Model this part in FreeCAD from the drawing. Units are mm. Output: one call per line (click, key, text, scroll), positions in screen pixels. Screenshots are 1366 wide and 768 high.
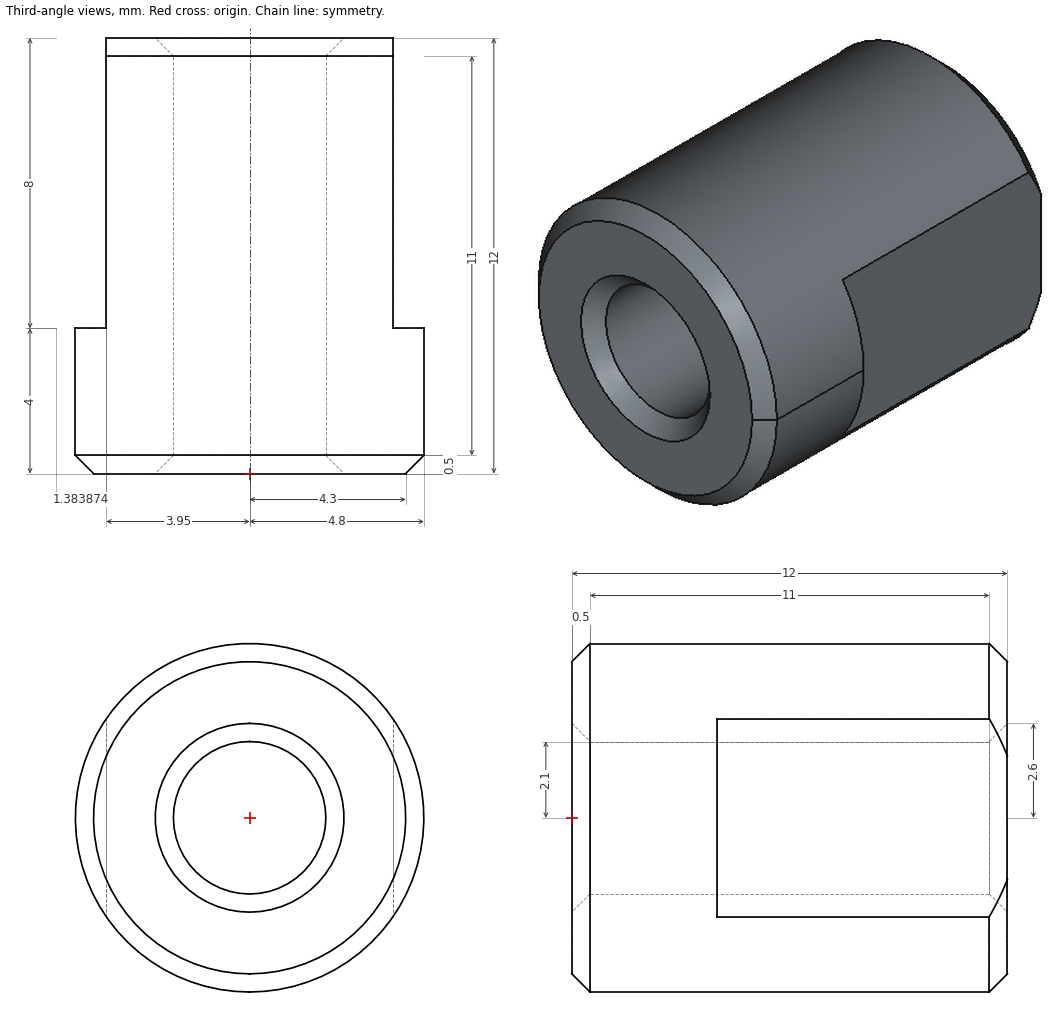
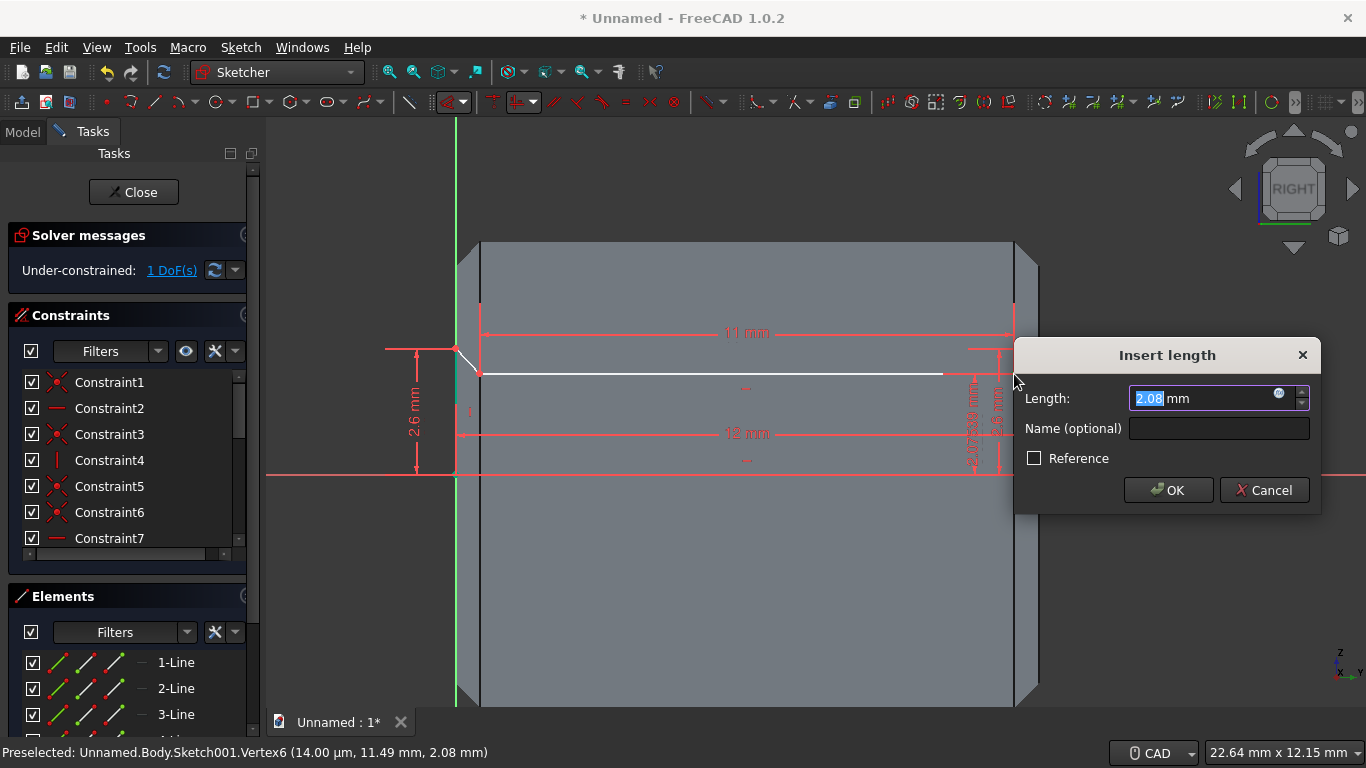
text(2.1)
key(Return)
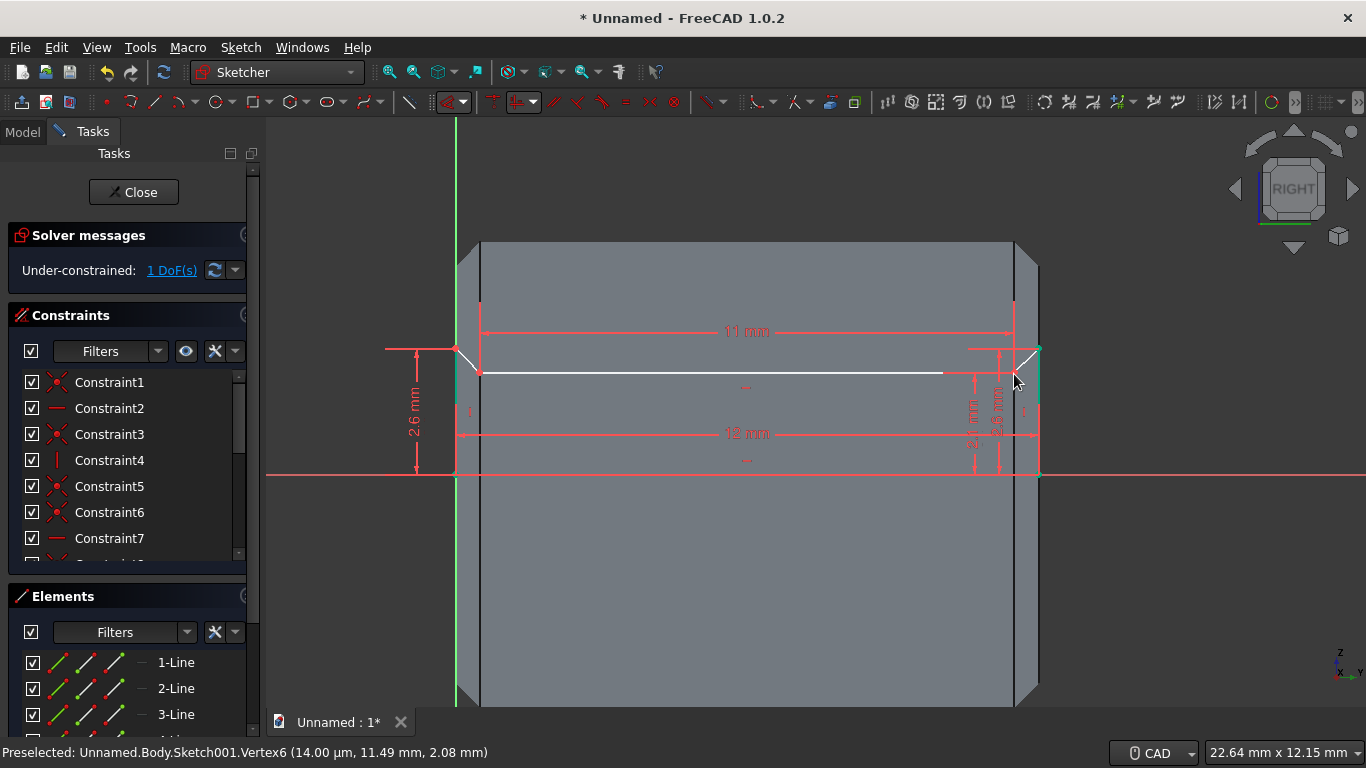
scroll(480, 373, up, 3)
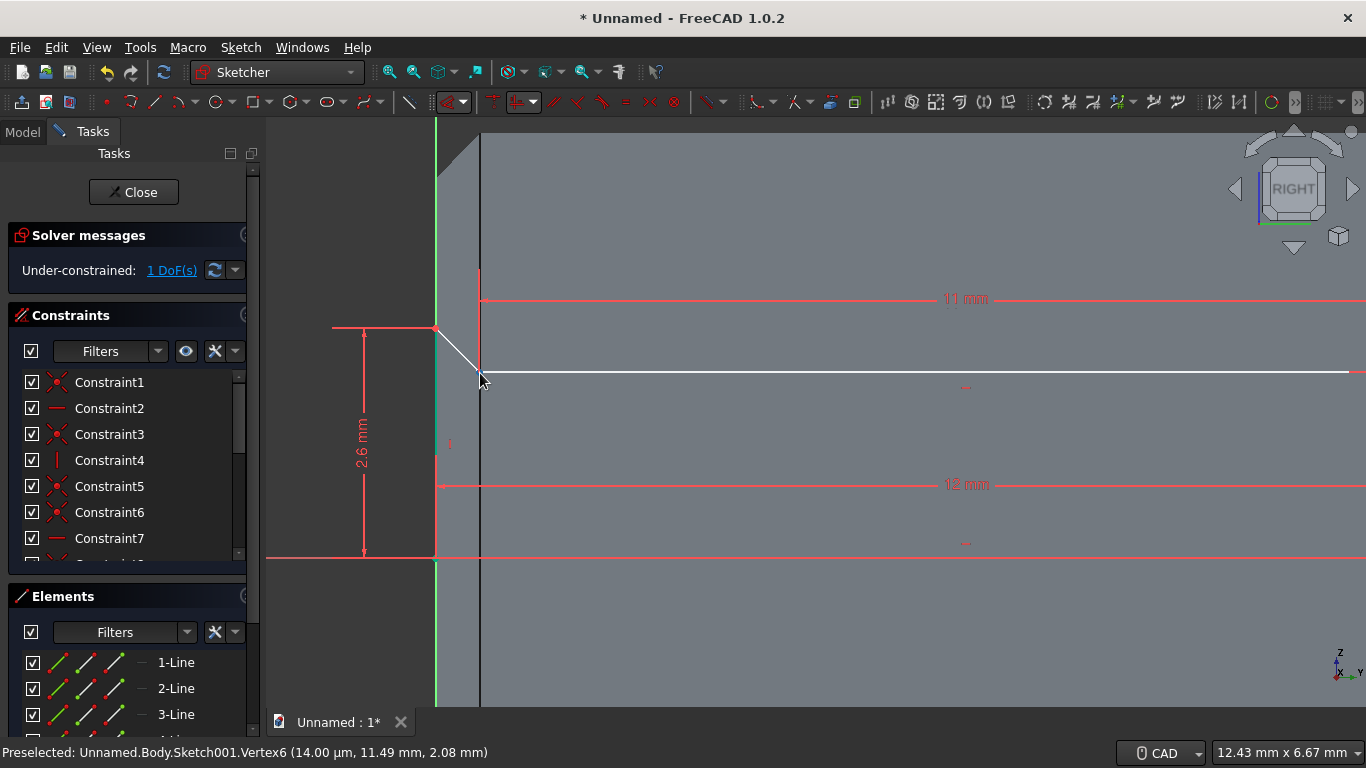
click(479, 372)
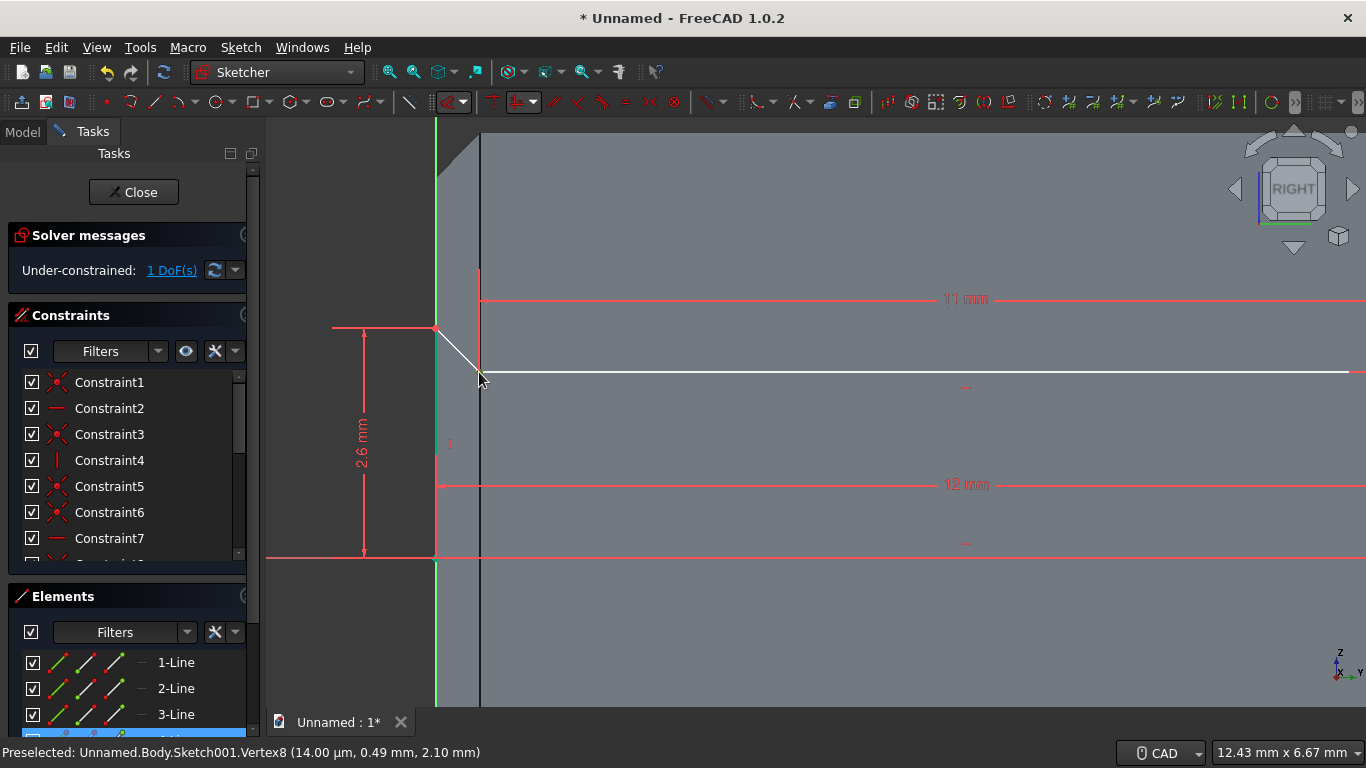
click(466, 102)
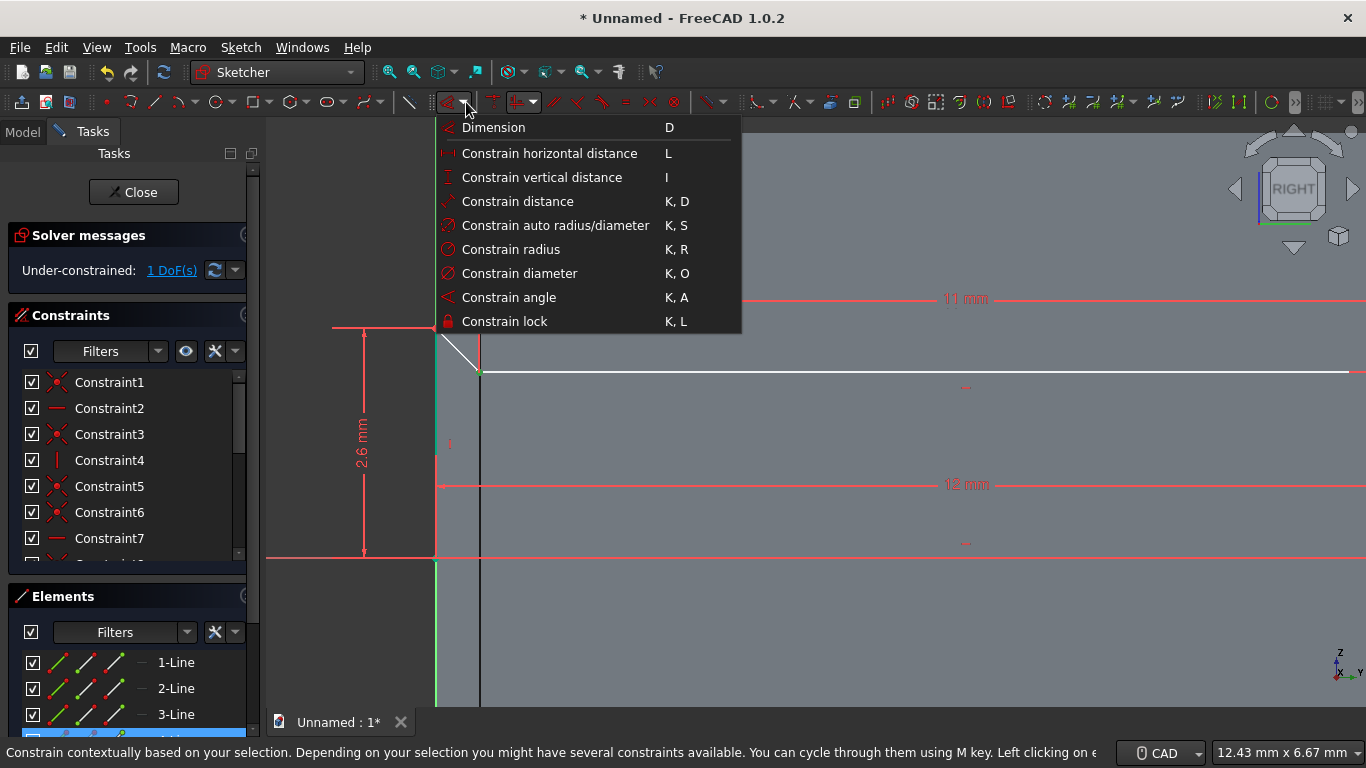
click(589, 153)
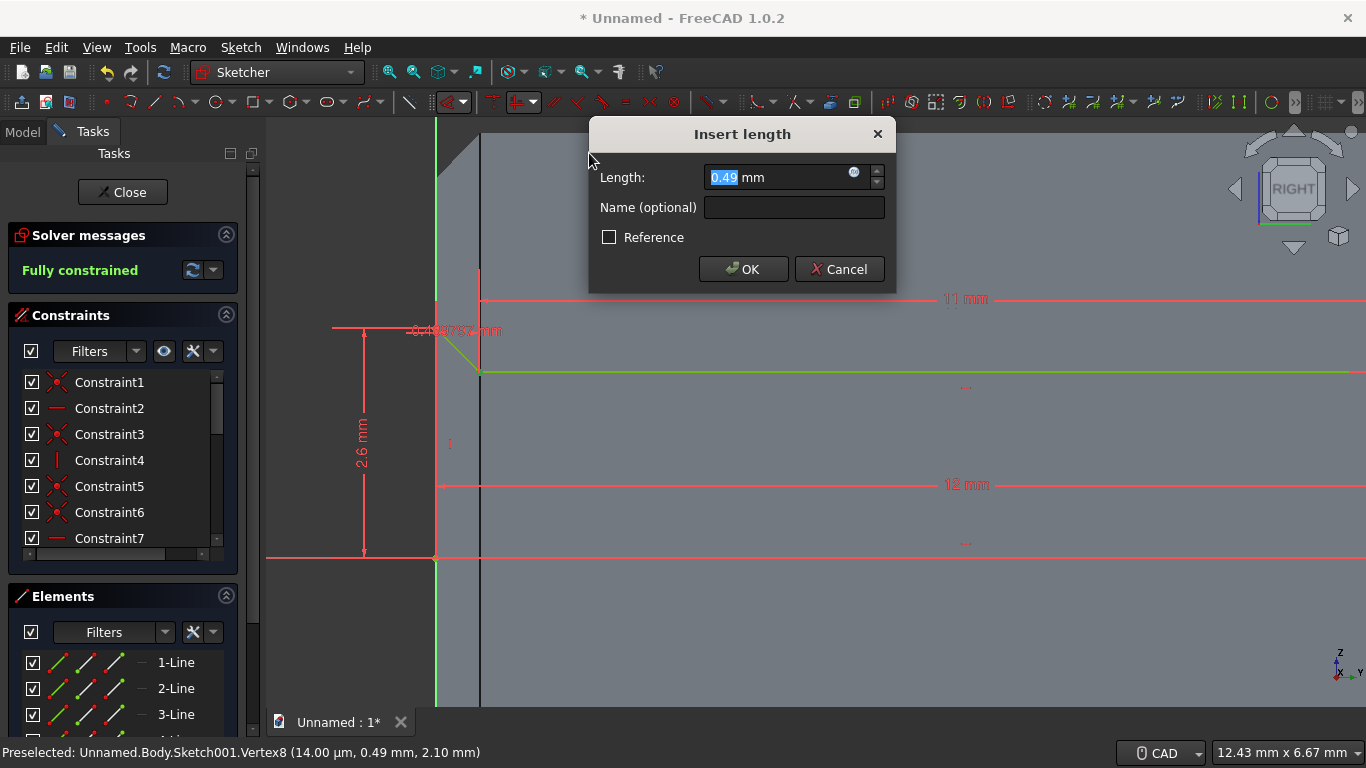
text(0.5)
key(Return)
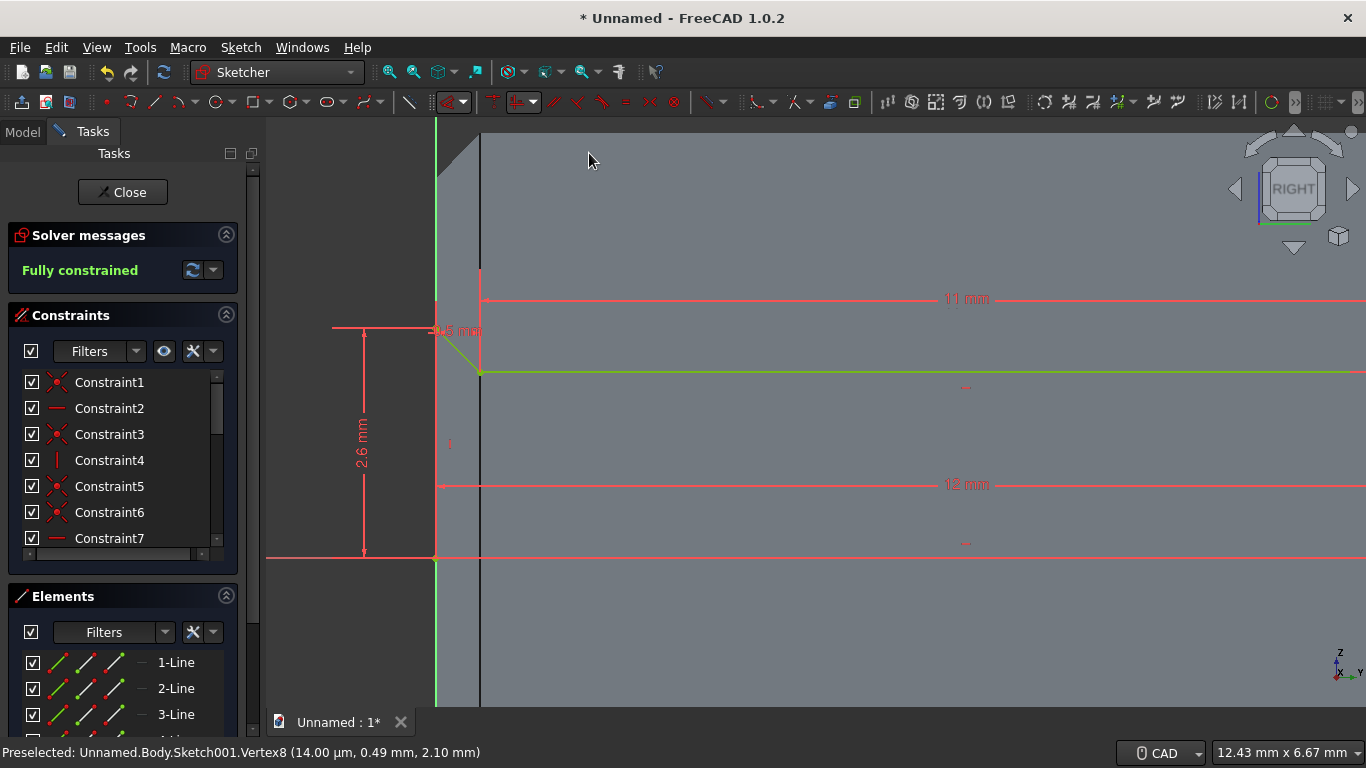
click(123, 192)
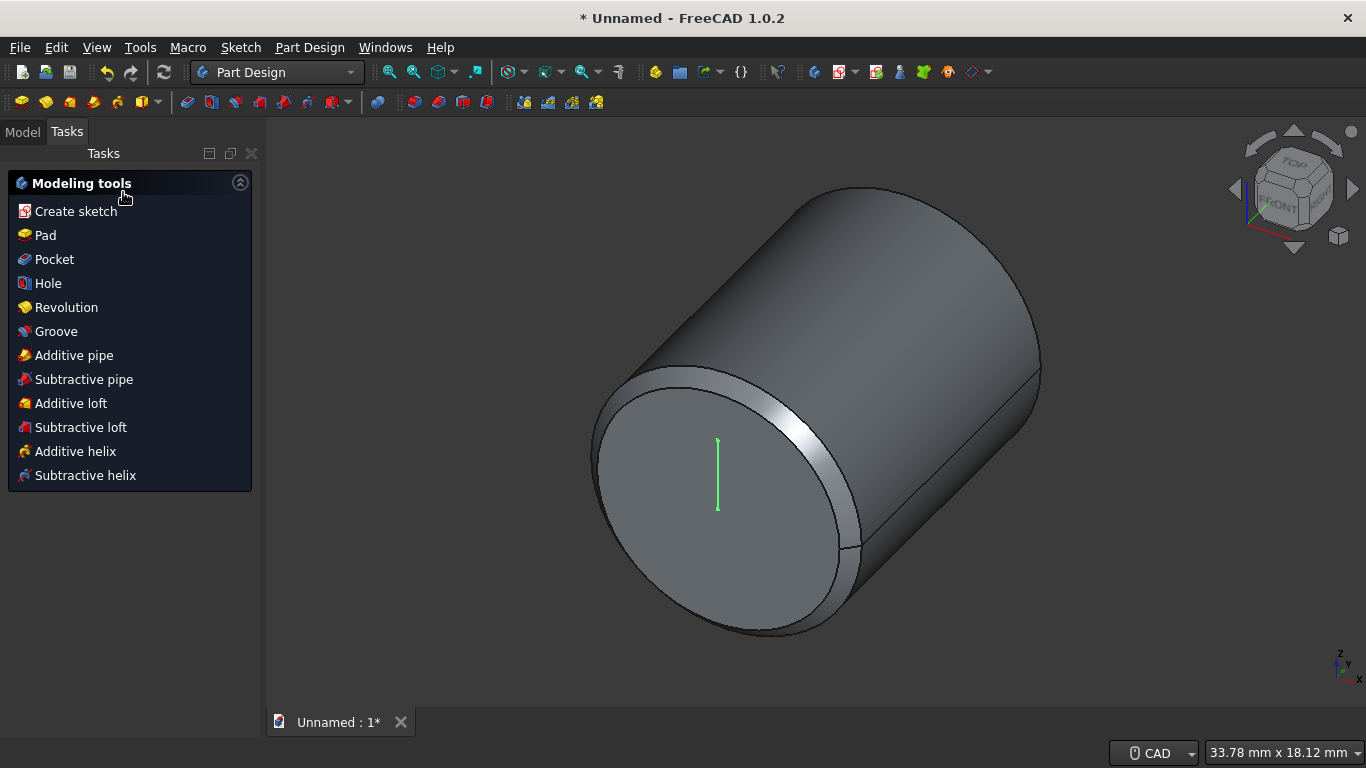
click(236, 102)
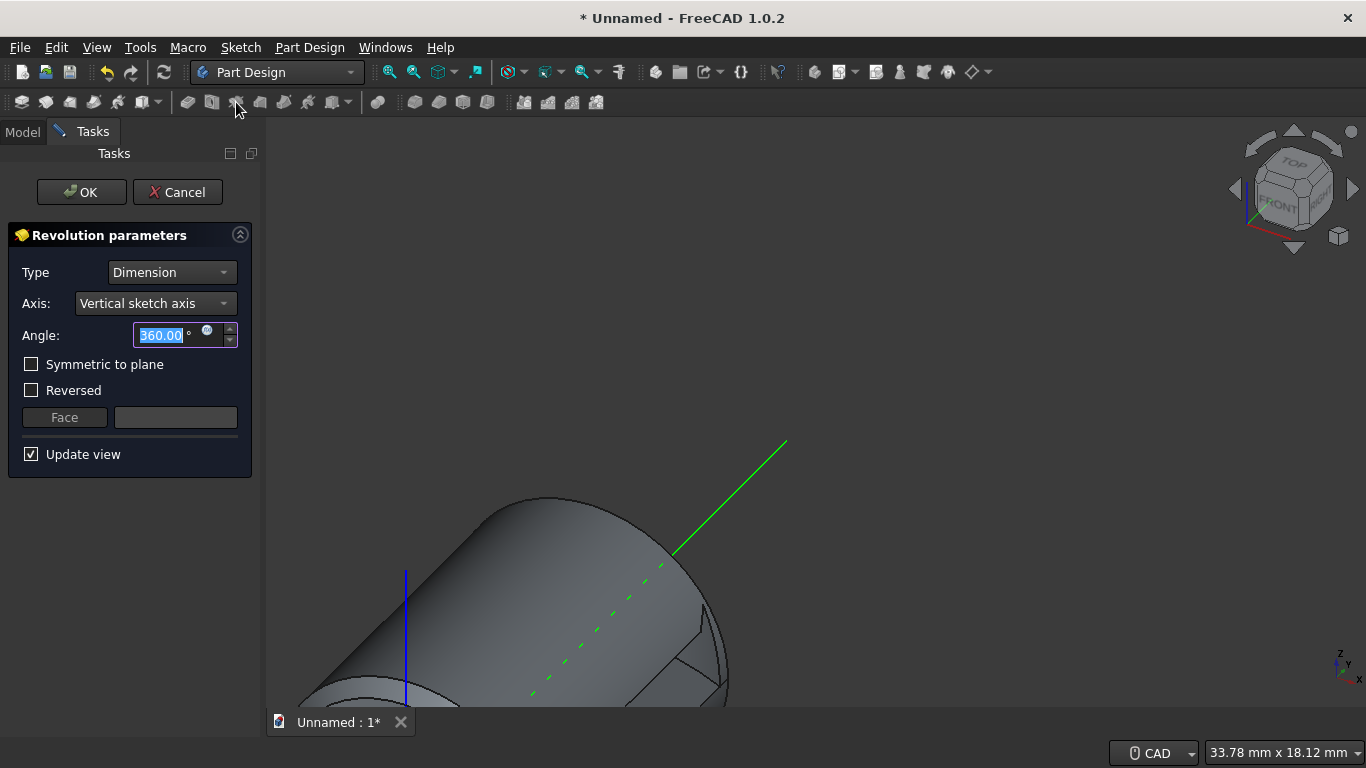
click(156, 304)